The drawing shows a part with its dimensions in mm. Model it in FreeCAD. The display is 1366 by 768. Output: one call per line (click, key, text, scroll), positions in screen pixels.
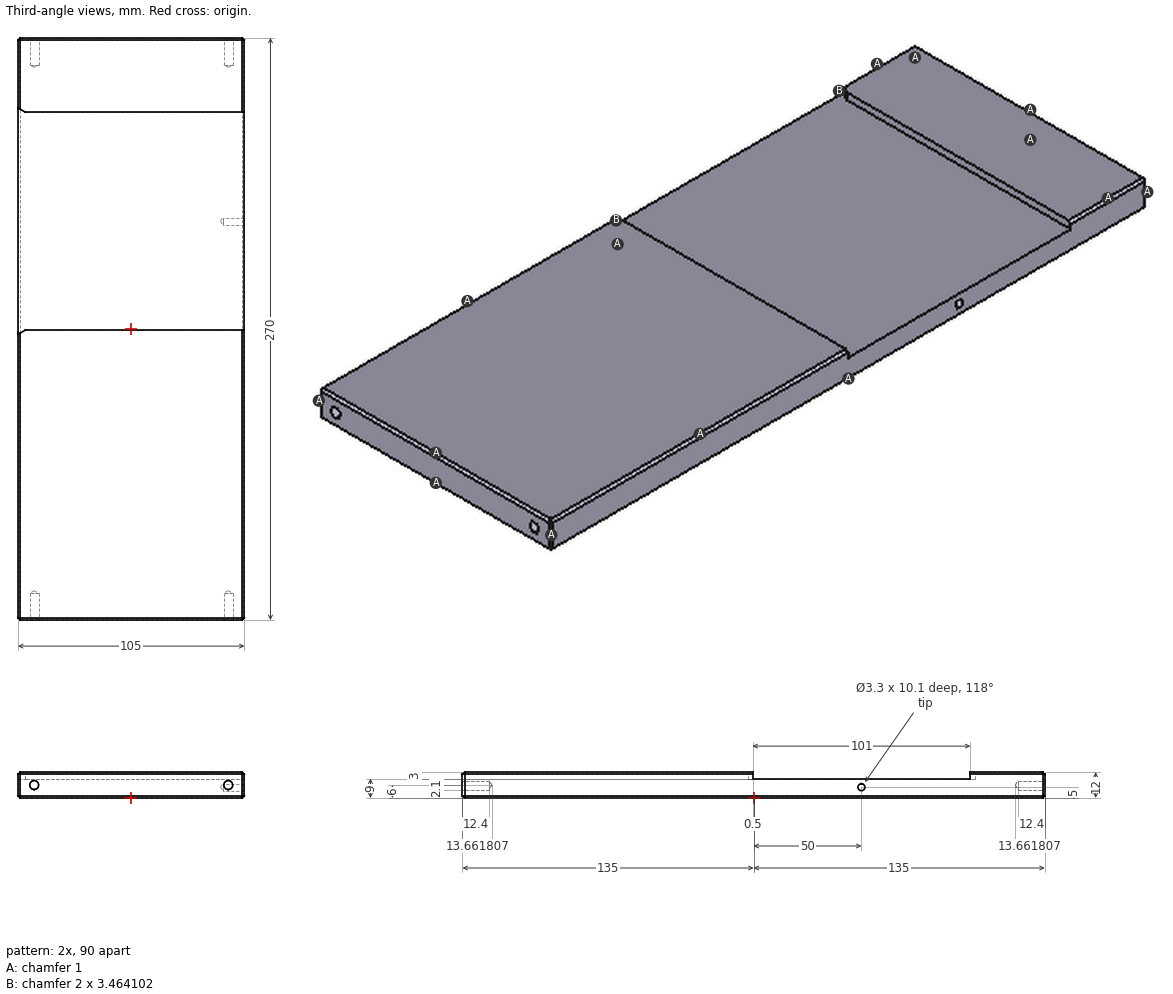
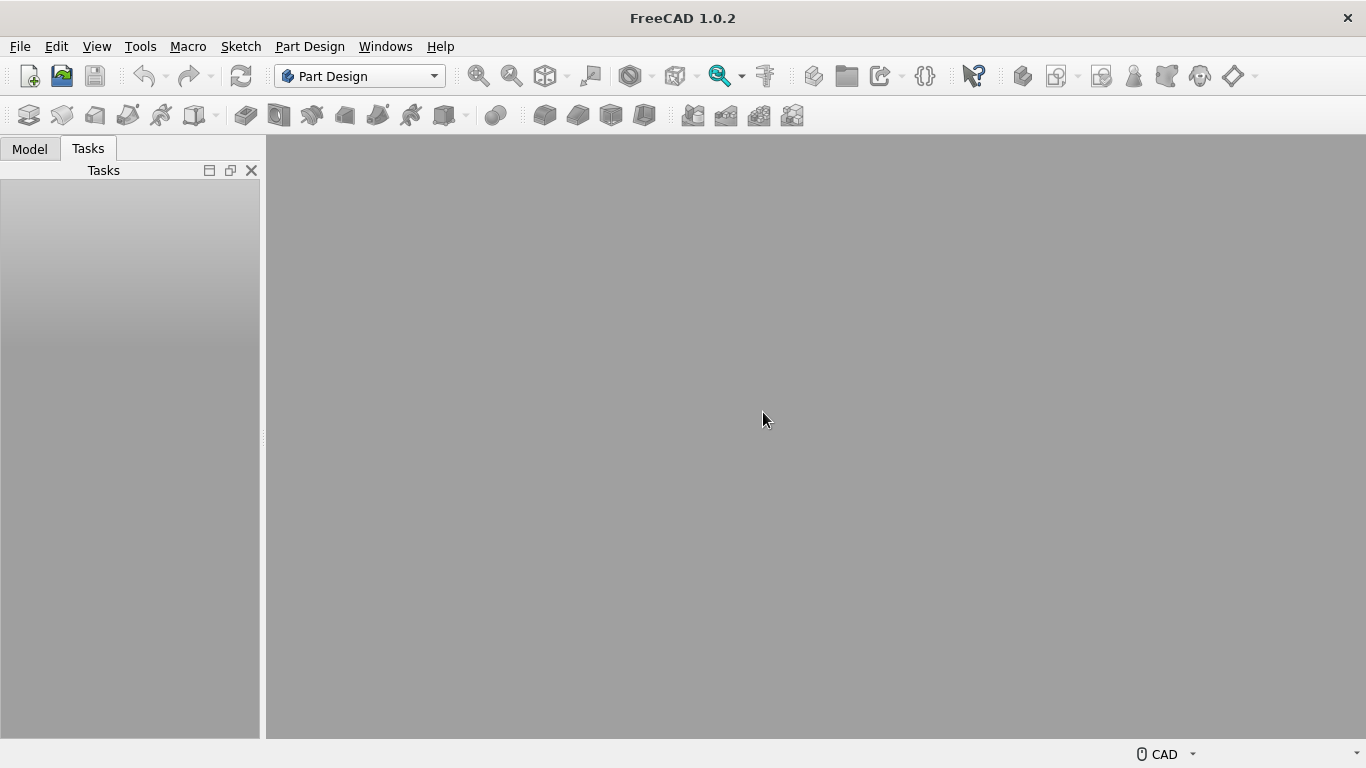
click(29, 76)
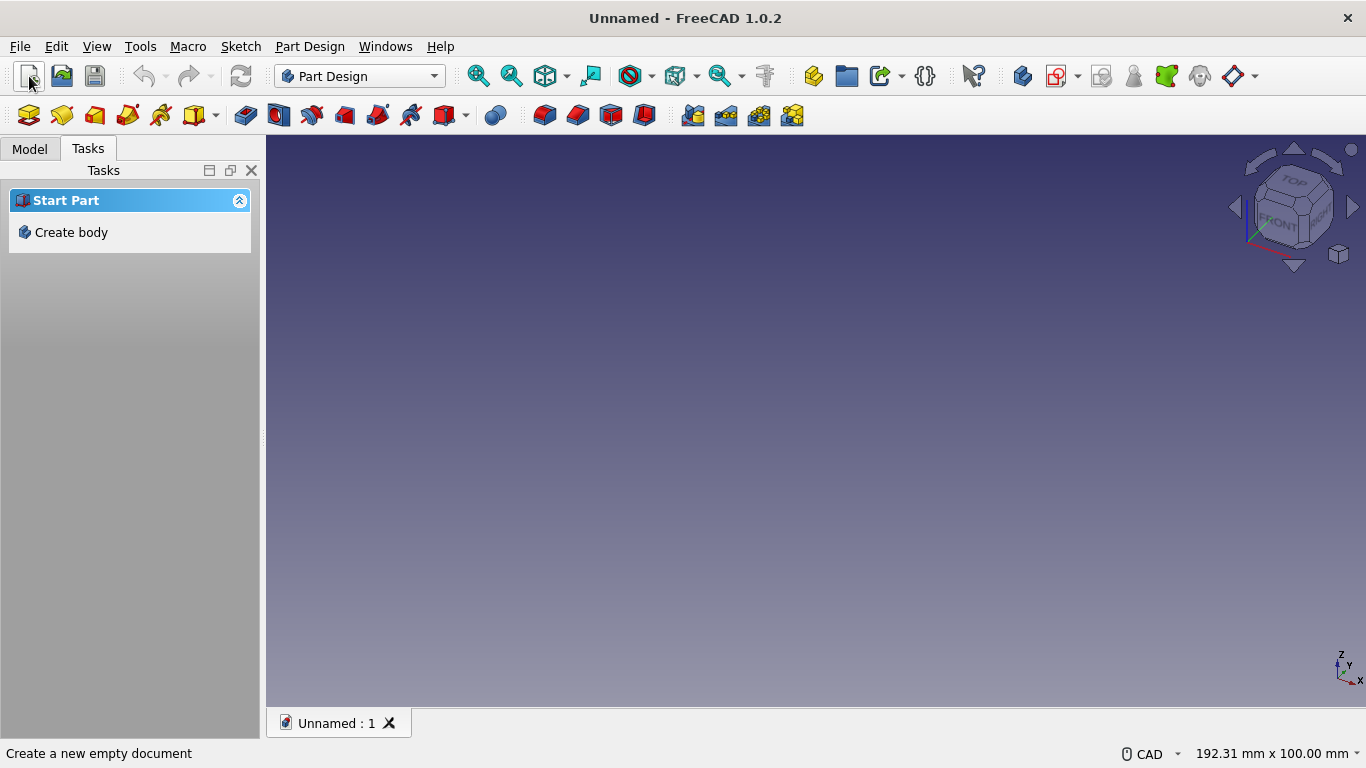
click(1056, 76)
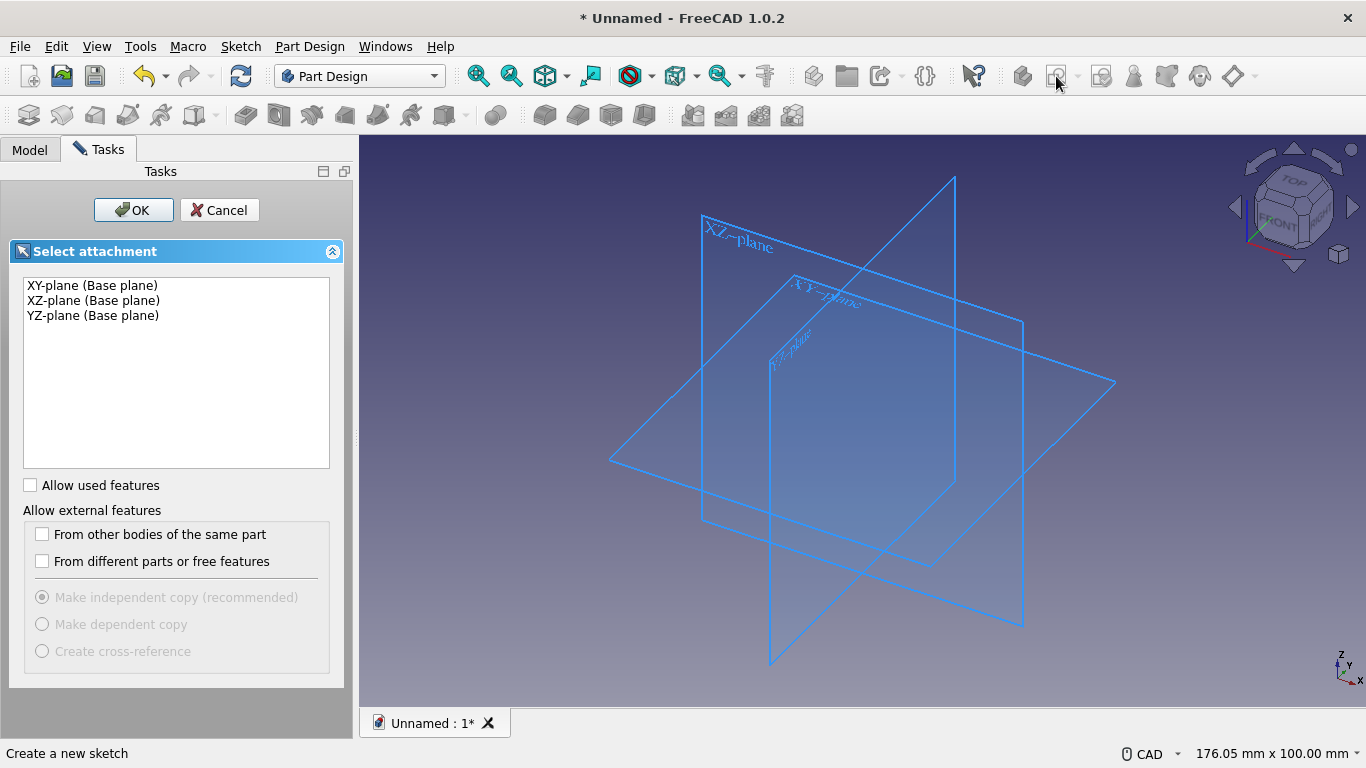
click(84, 286)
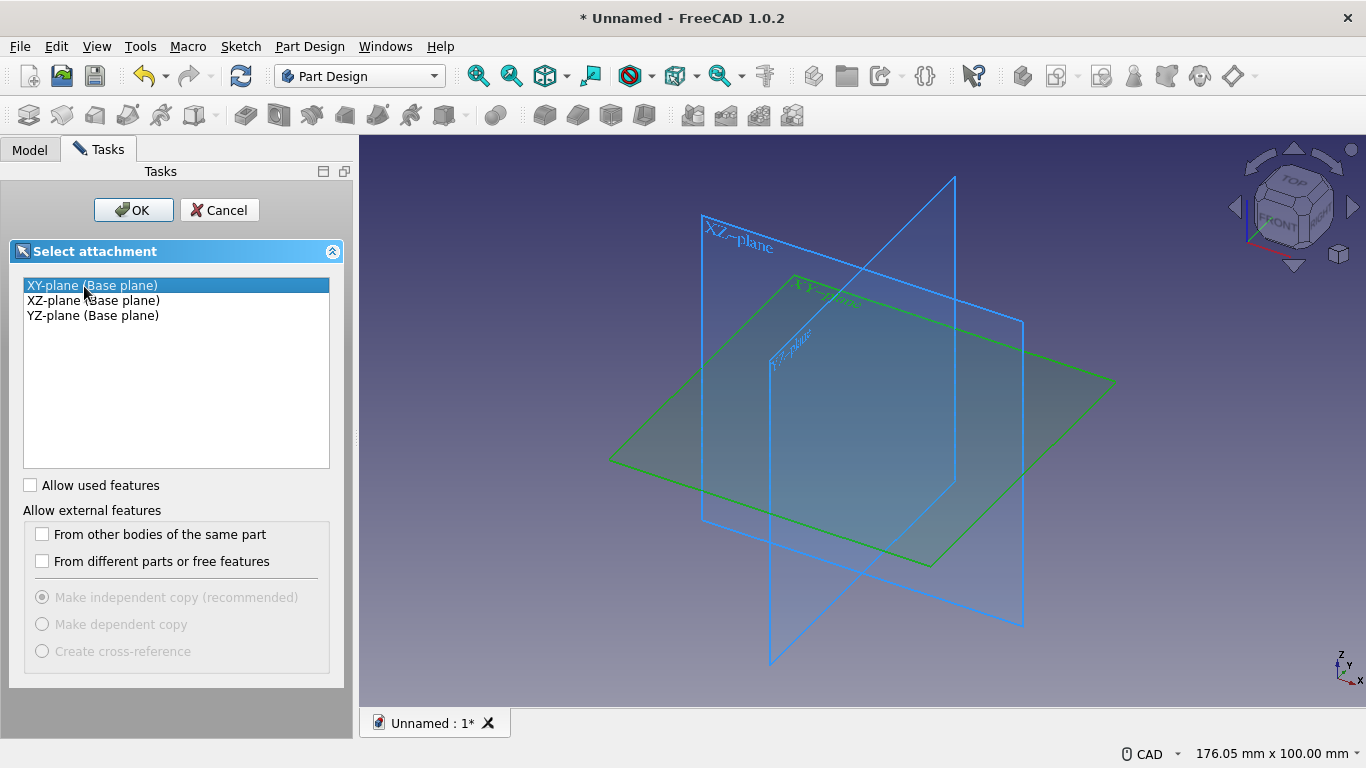
click(134, 210)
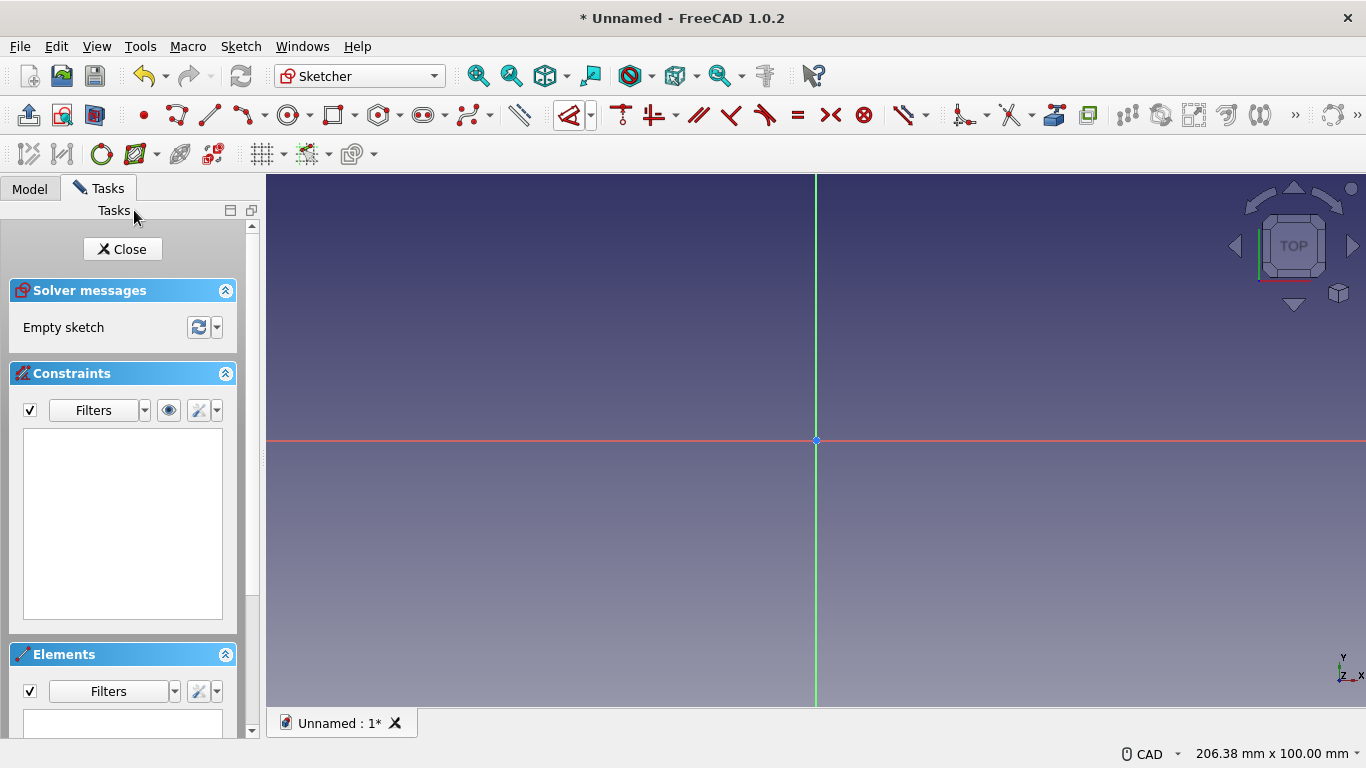
scroll(725, 440, down, 7)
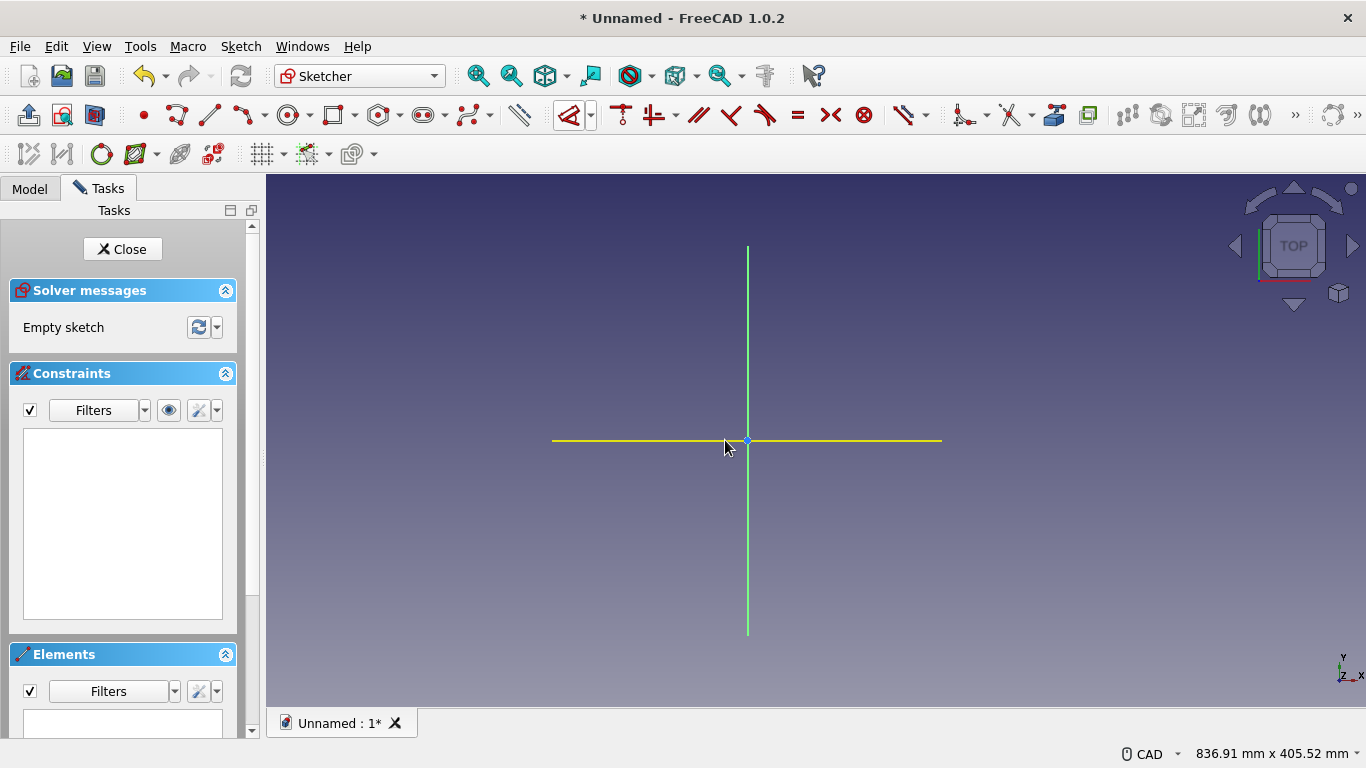
click(354, 116)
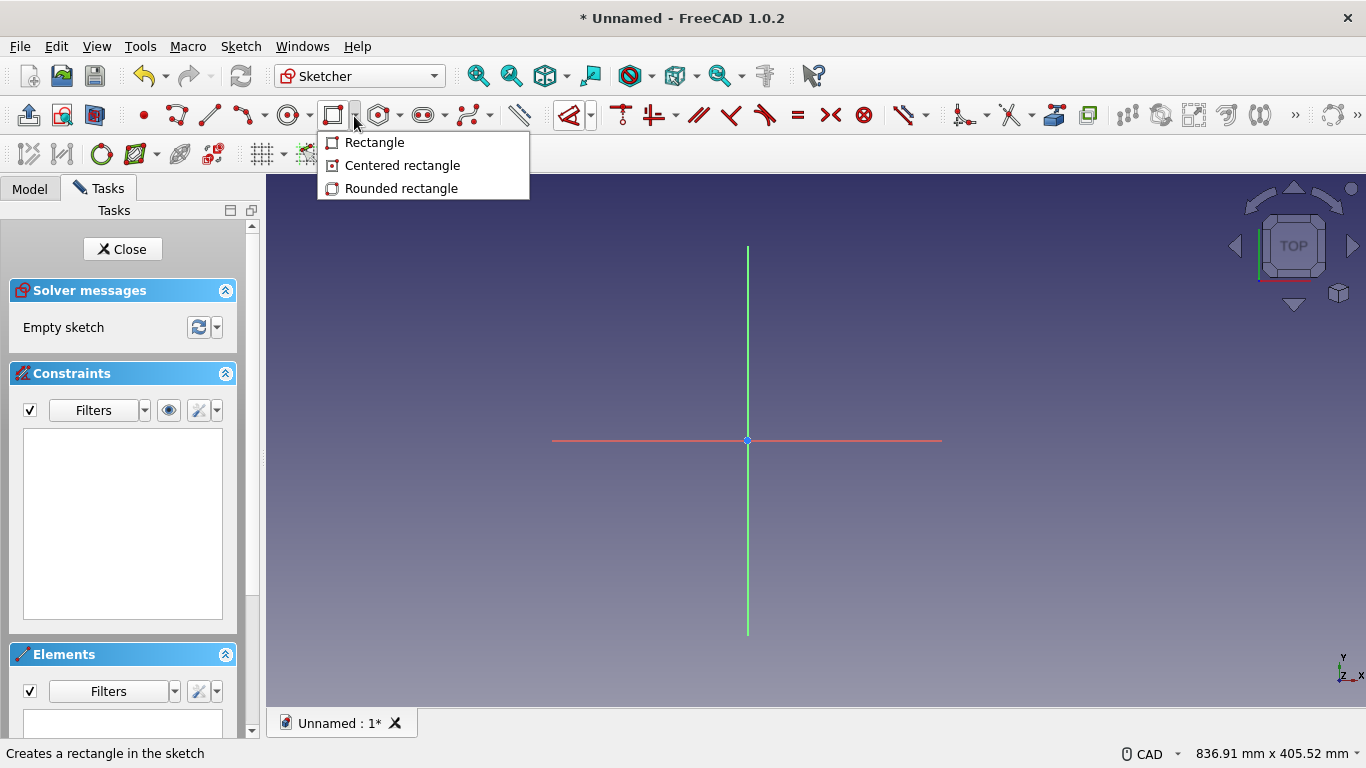
click(424, 166)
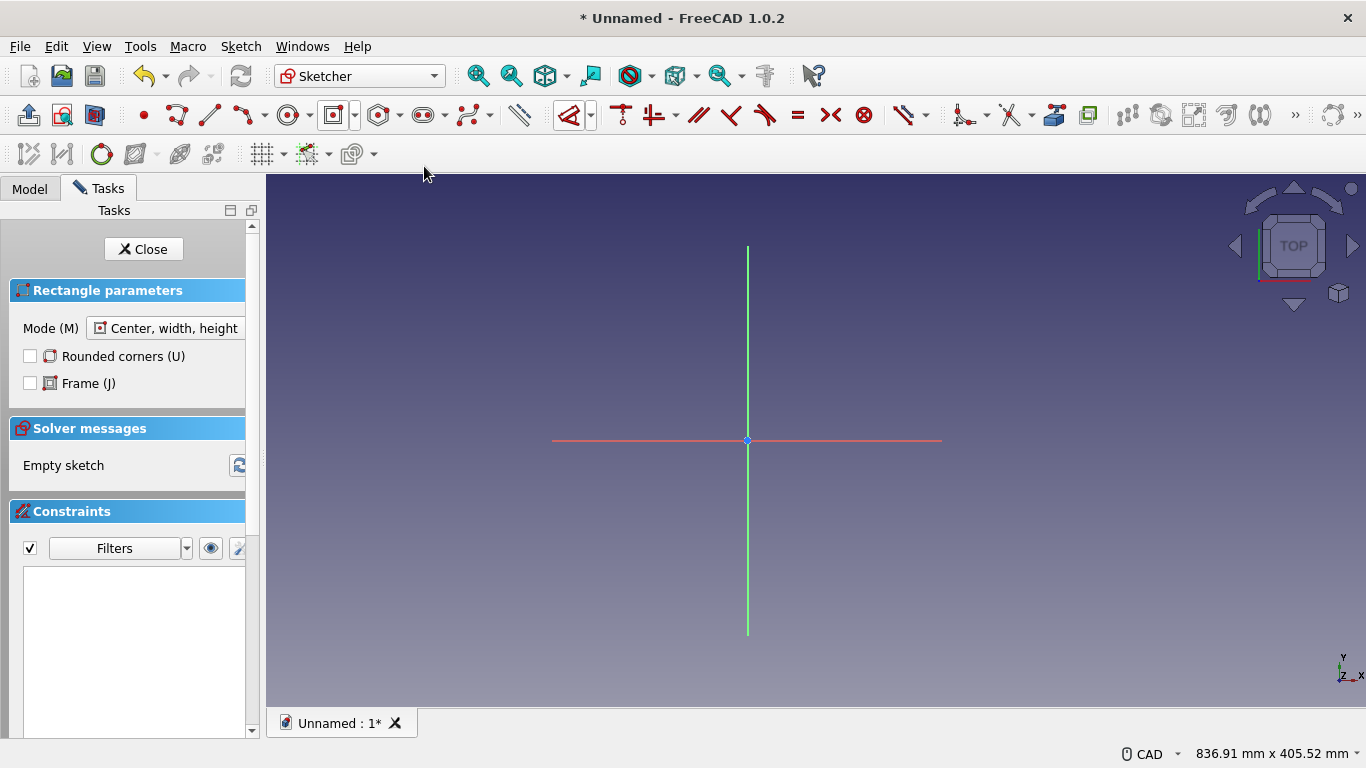
click(748, 440)
move(817, 263)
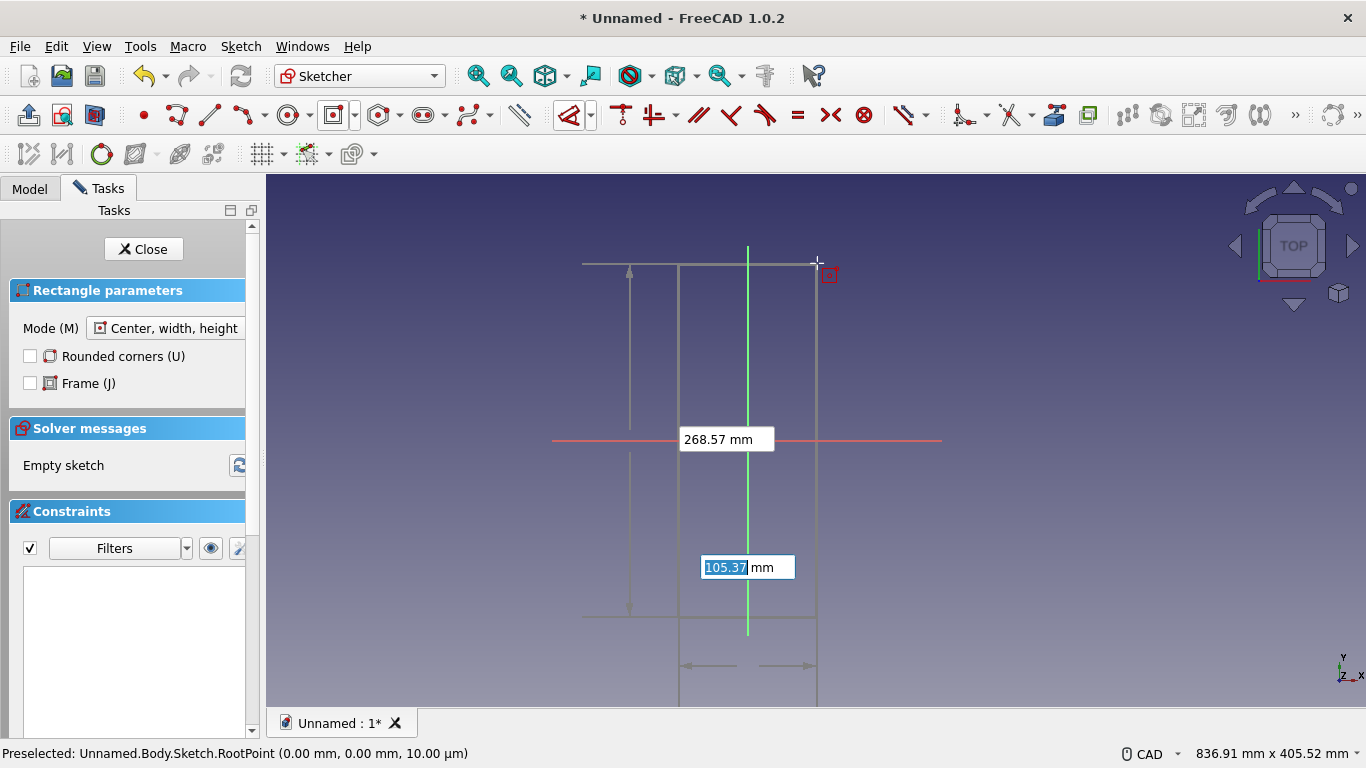
text(105)
key(Tab)
text(270)
key(Return)
key(Escape)